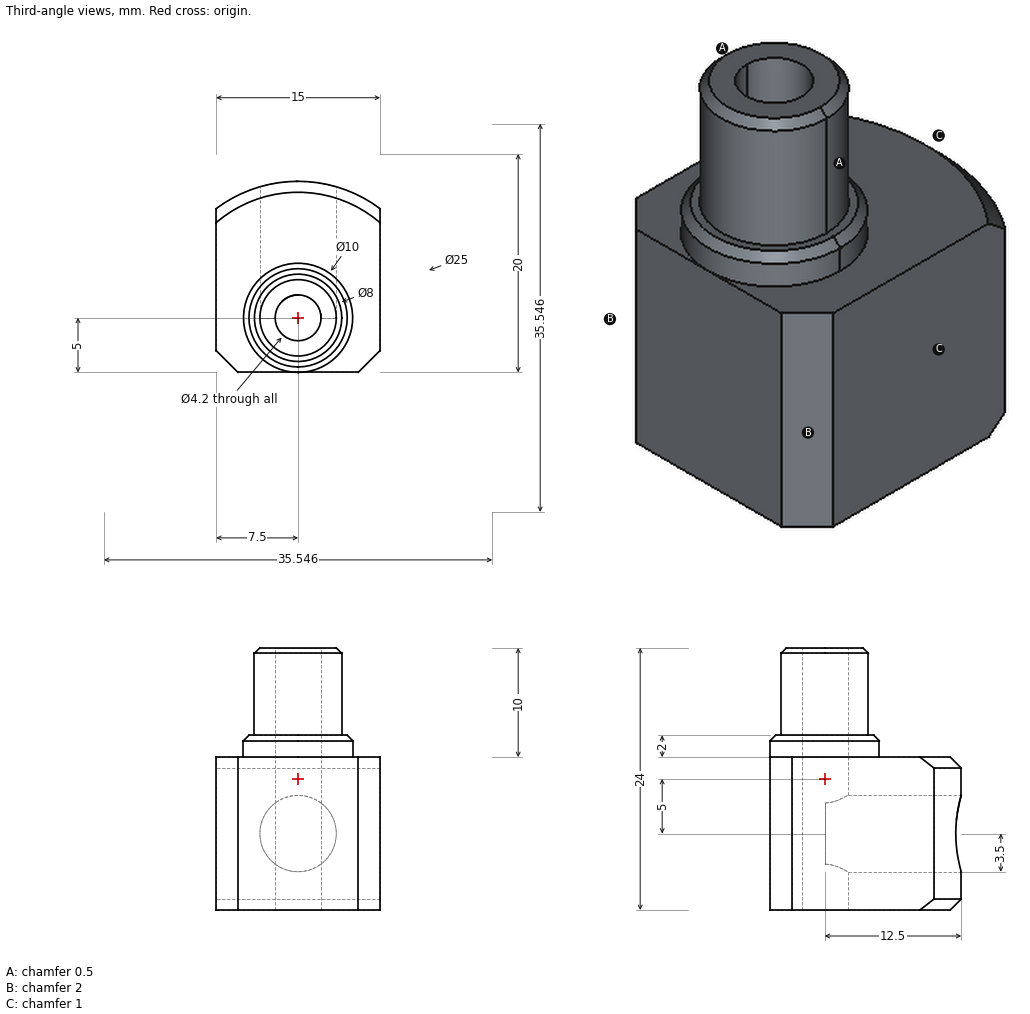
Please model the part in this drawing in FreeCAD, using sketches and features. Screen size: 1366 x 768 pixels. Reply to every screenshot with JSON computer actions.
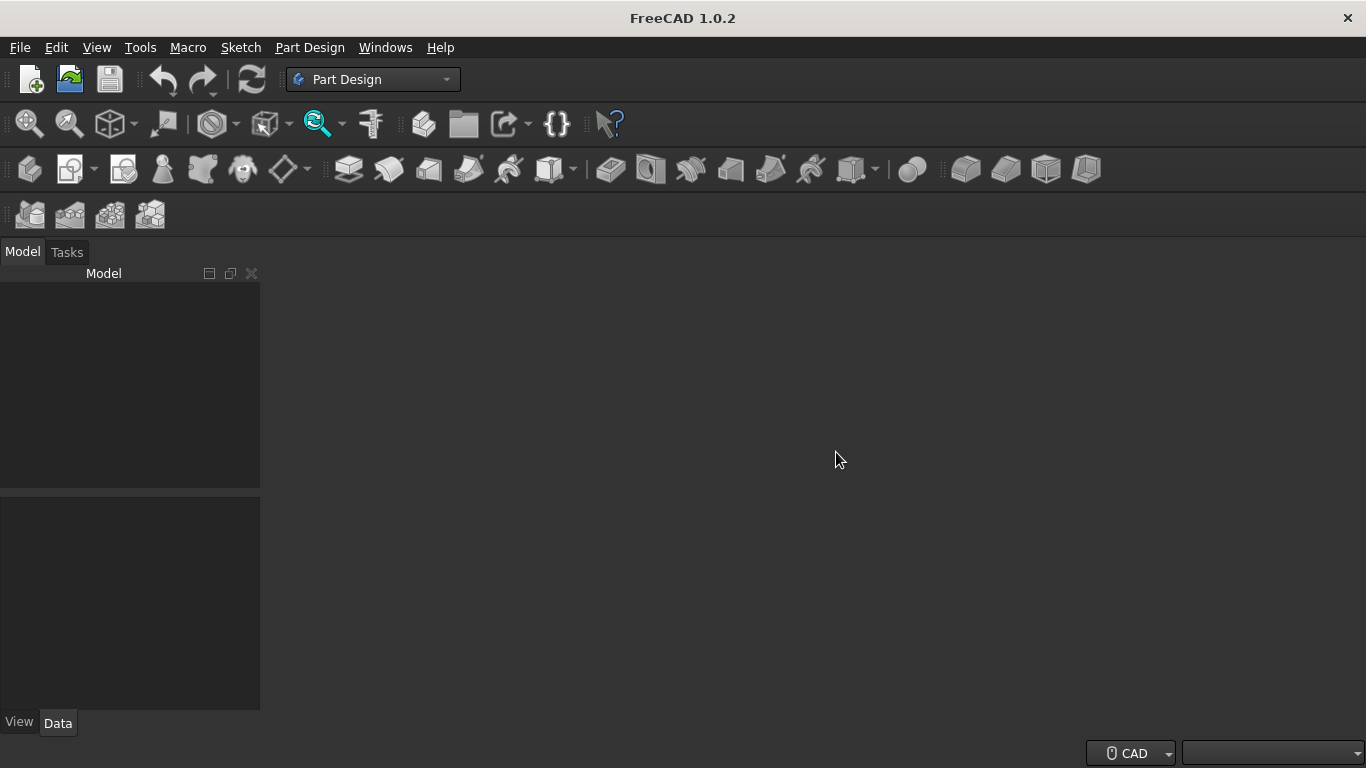
{"action": "left_click", "coordinate": [30, 80]}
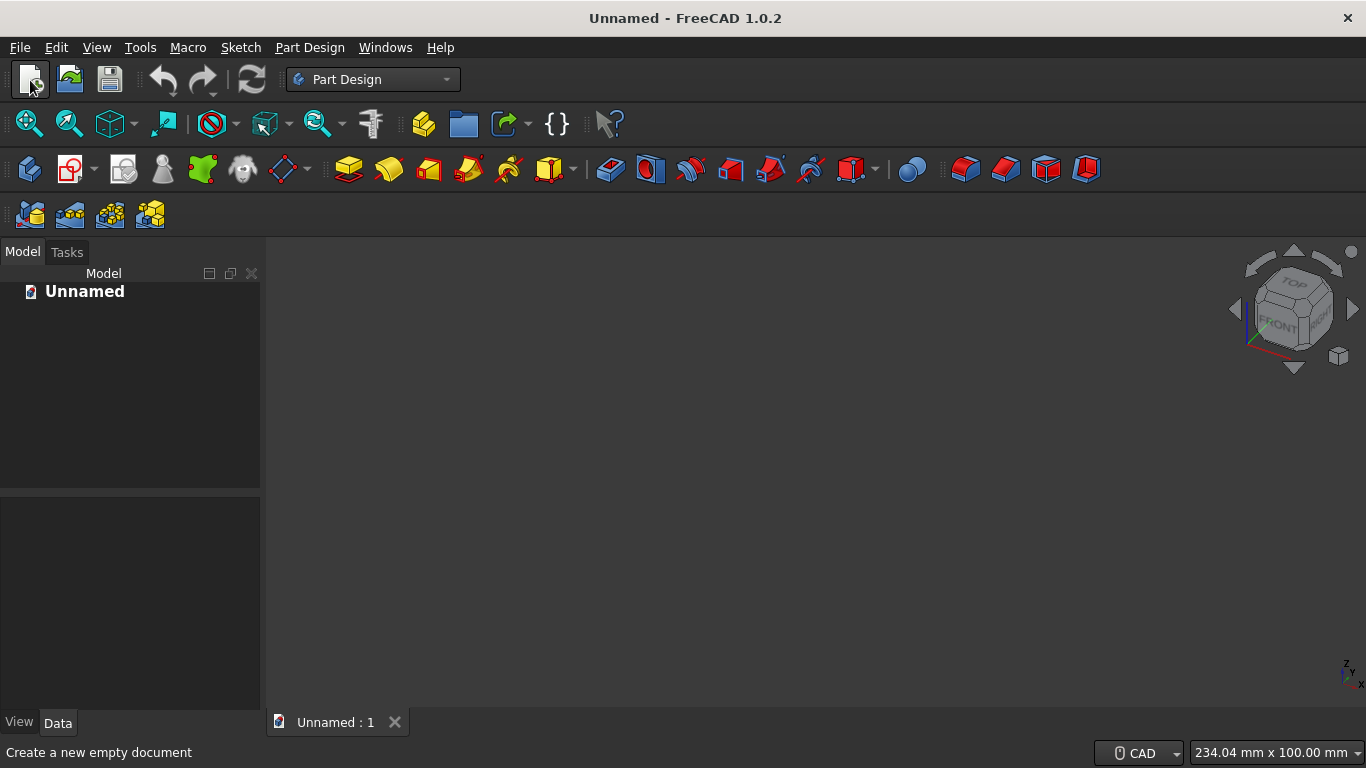
{"action": "left_click", "coordinate": [70, 170]}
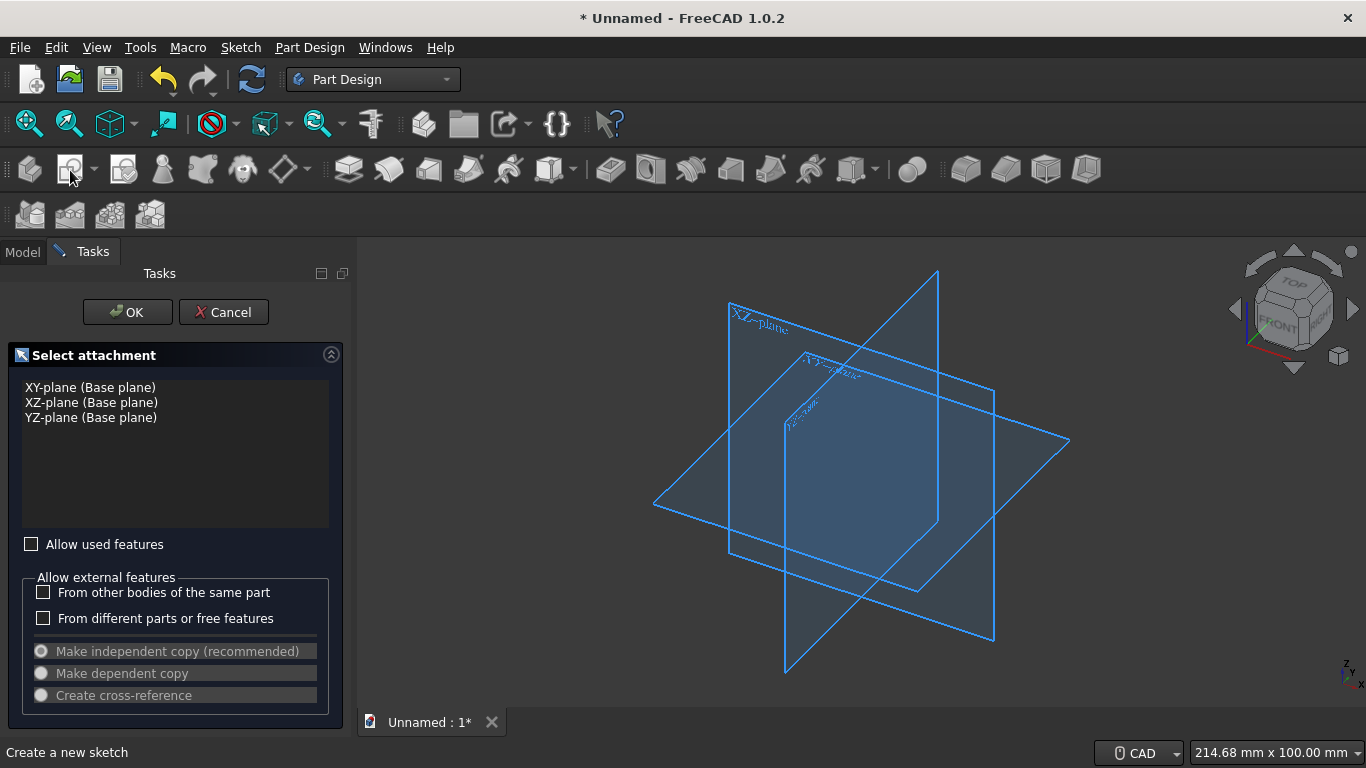
{"action": "left_click", "coordinate": [82, 388]}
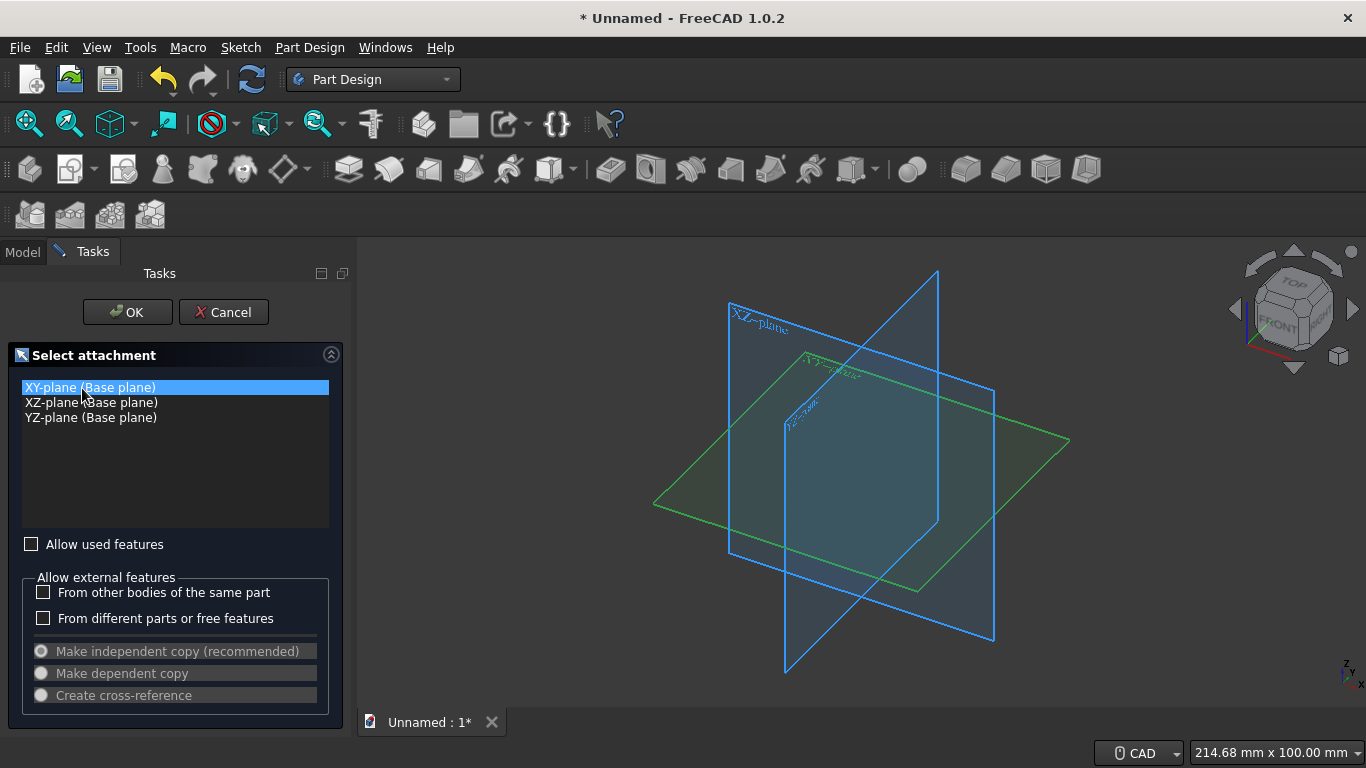
{"action": "left_click", "coordinate": [128, 312]}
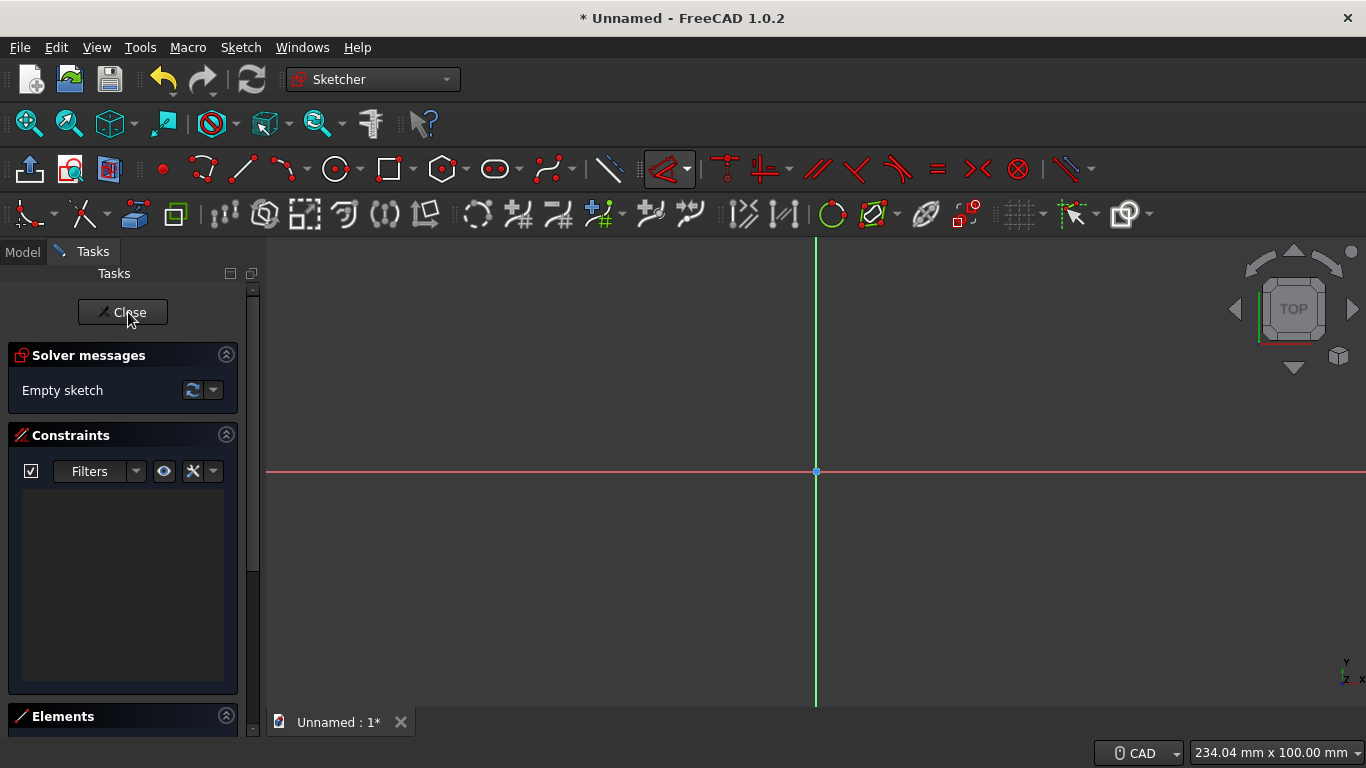
{"action": "scroll", "coordinate": [856, 472], "scroll_direction": "up", "scroll_amount": 5}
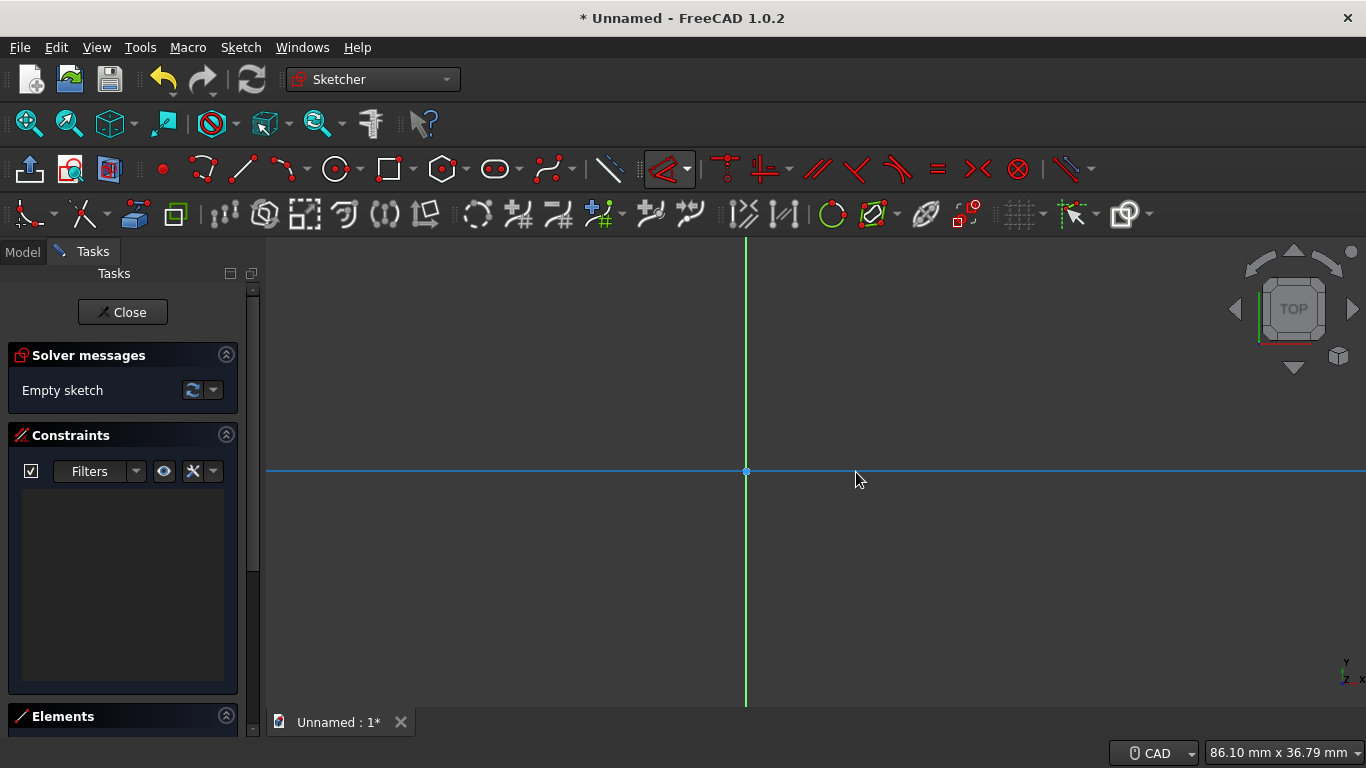
{"action": "left_click", "coordinate": [336, 170]}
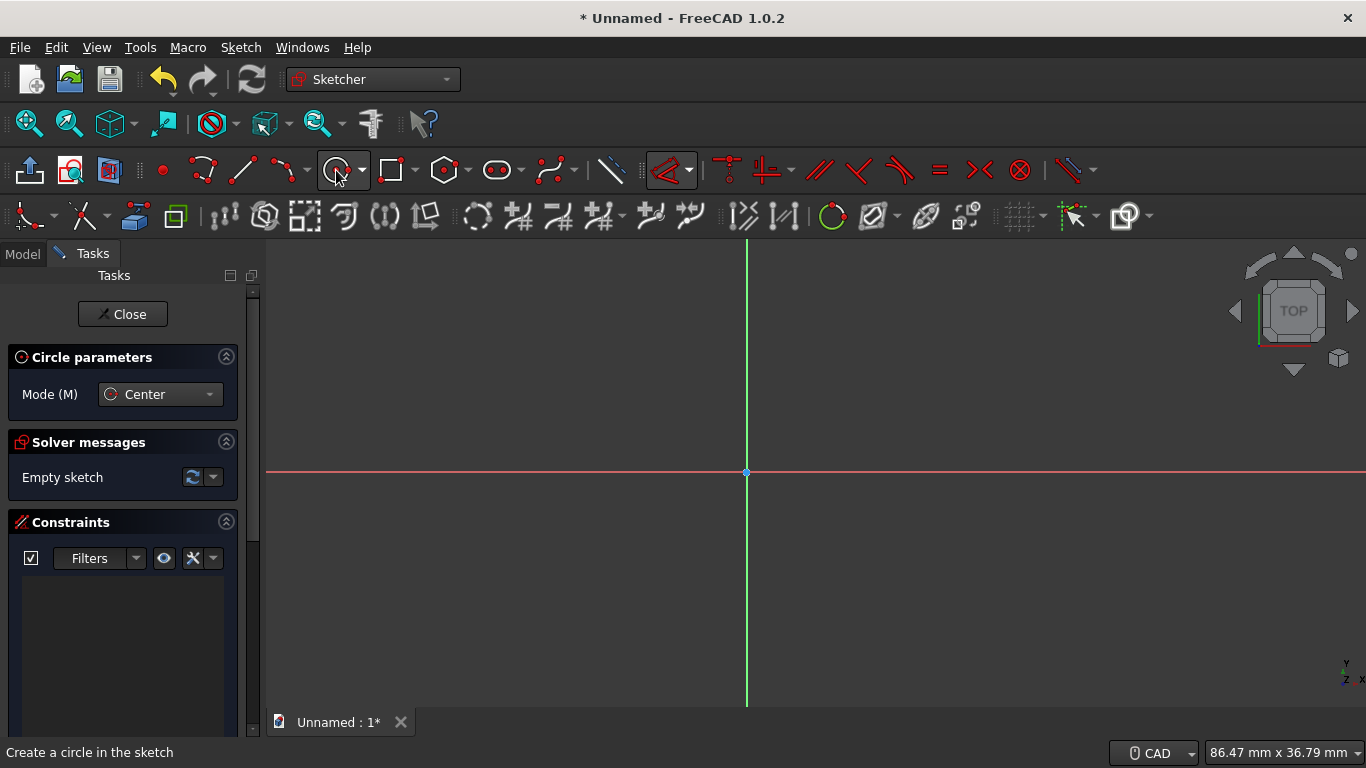
{"action": "left_click", "coordinate": [747, 472]}
{"action": "mouse_move", "coordinate": [859, 360]}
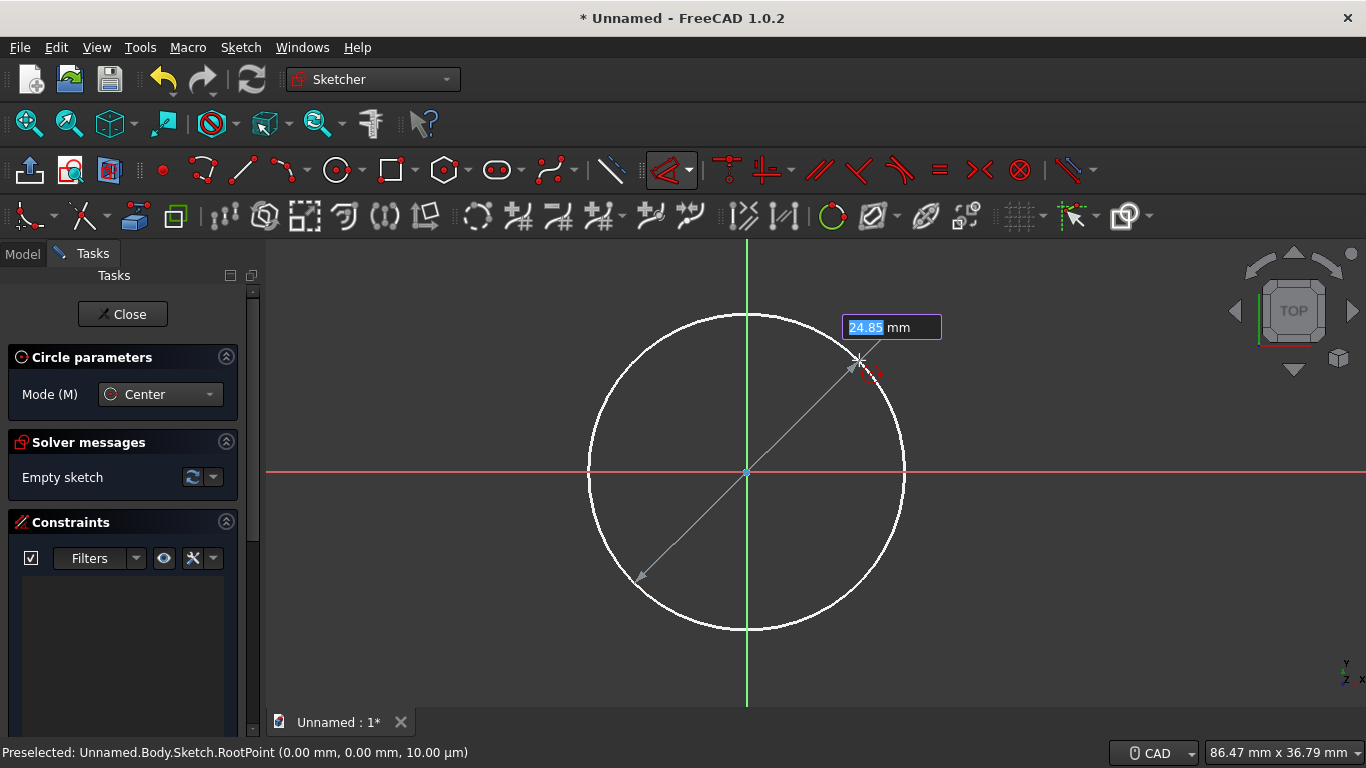
{"action": "type", "text": "25"}
{"action": "key", "text": "Return"}
{"action": "key", "text": "Escape"}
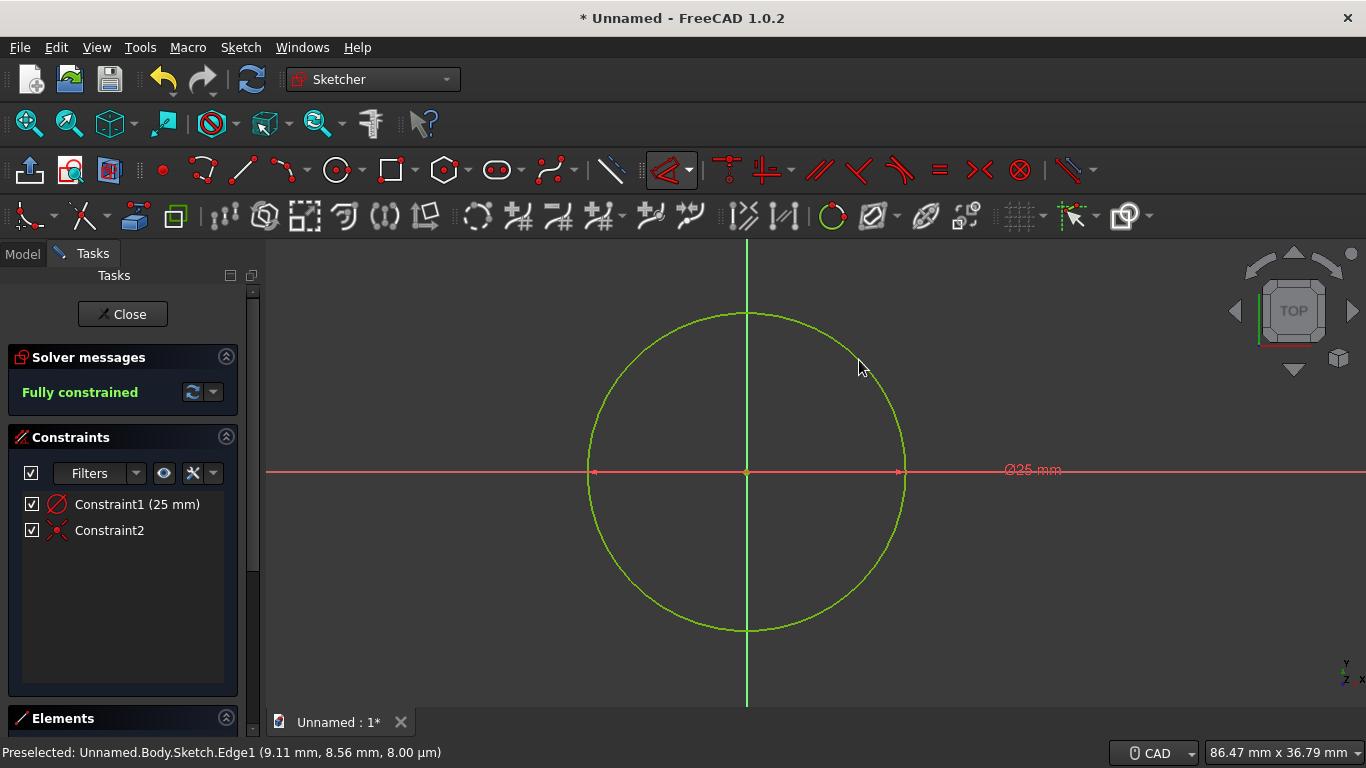
{"action": "left_click", "coordinate": [123, 314]}